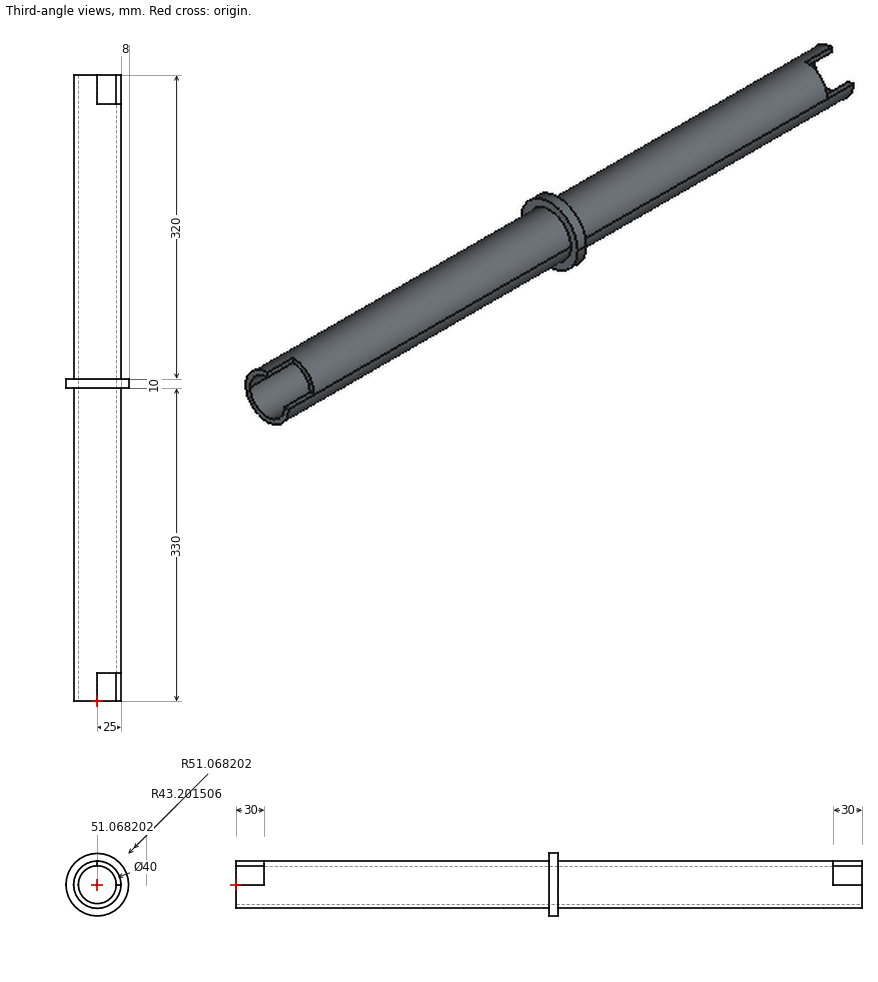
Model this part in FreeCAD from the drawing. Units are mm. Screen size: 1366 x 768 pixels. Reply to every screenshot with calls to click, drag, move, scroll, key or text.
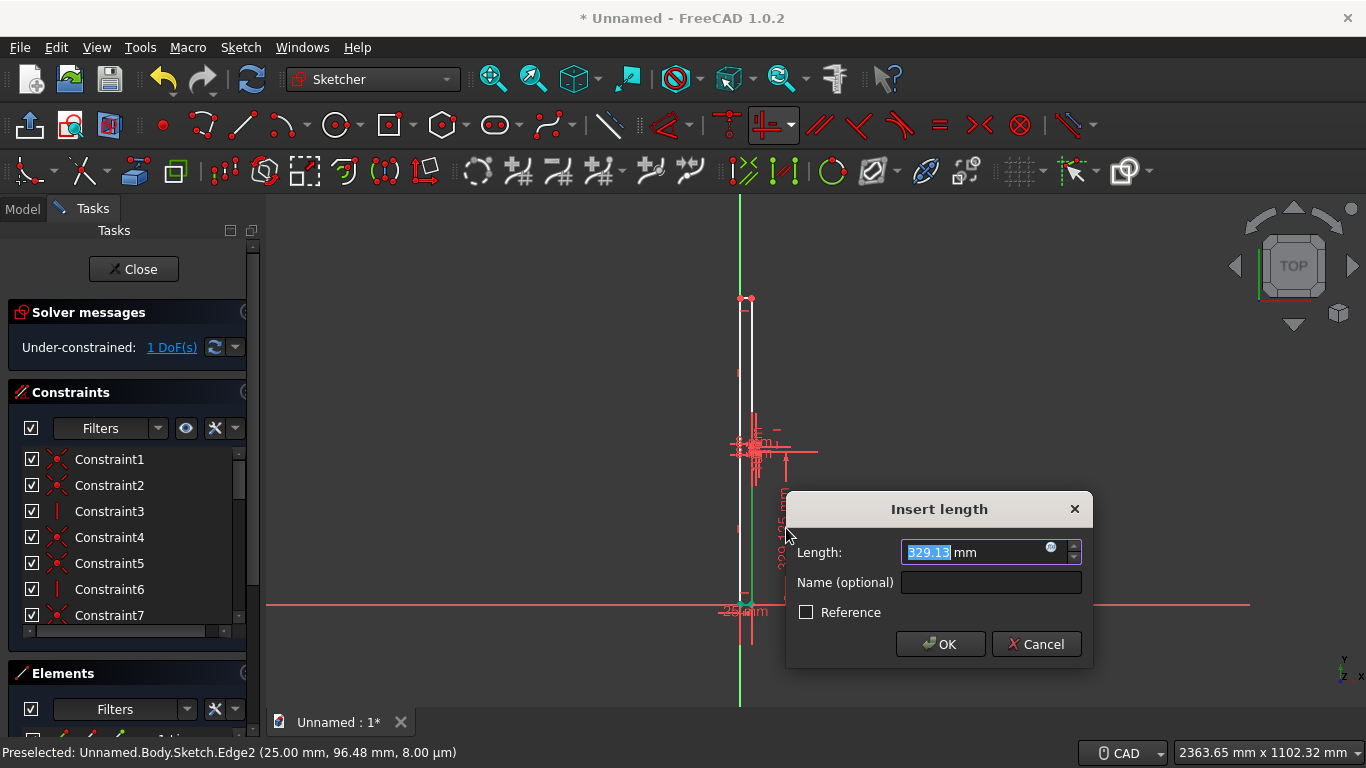
text(330)
key(Return)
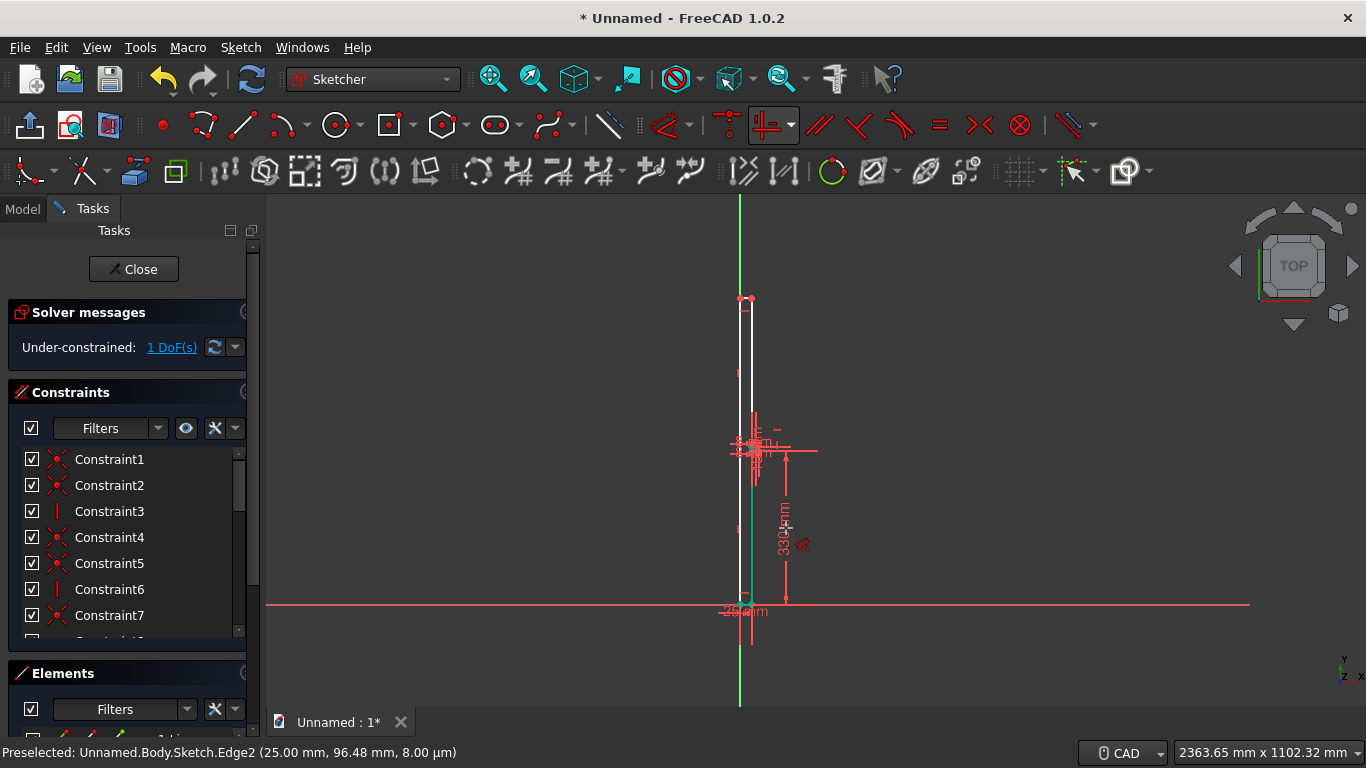
click(752, 402)
click(786, 372)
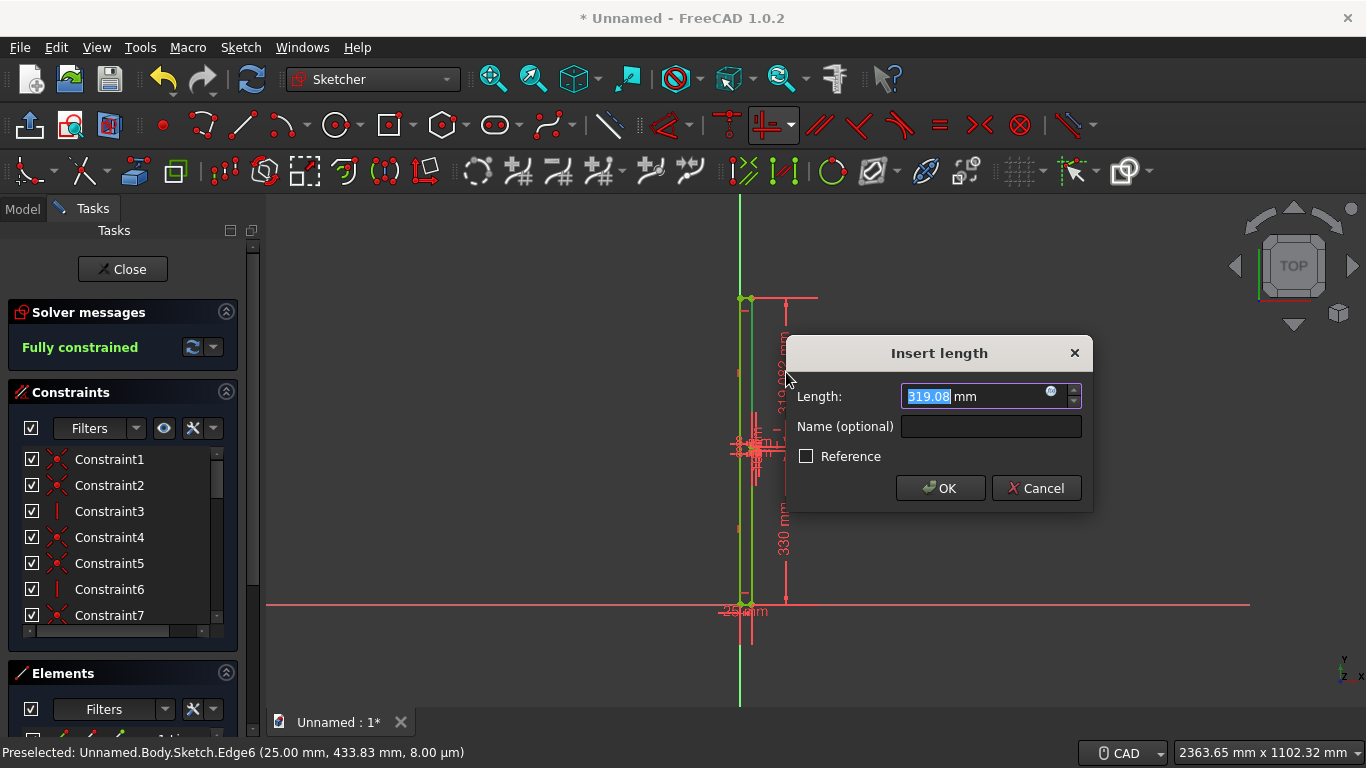
text(320)
key(Return)
key(Escape)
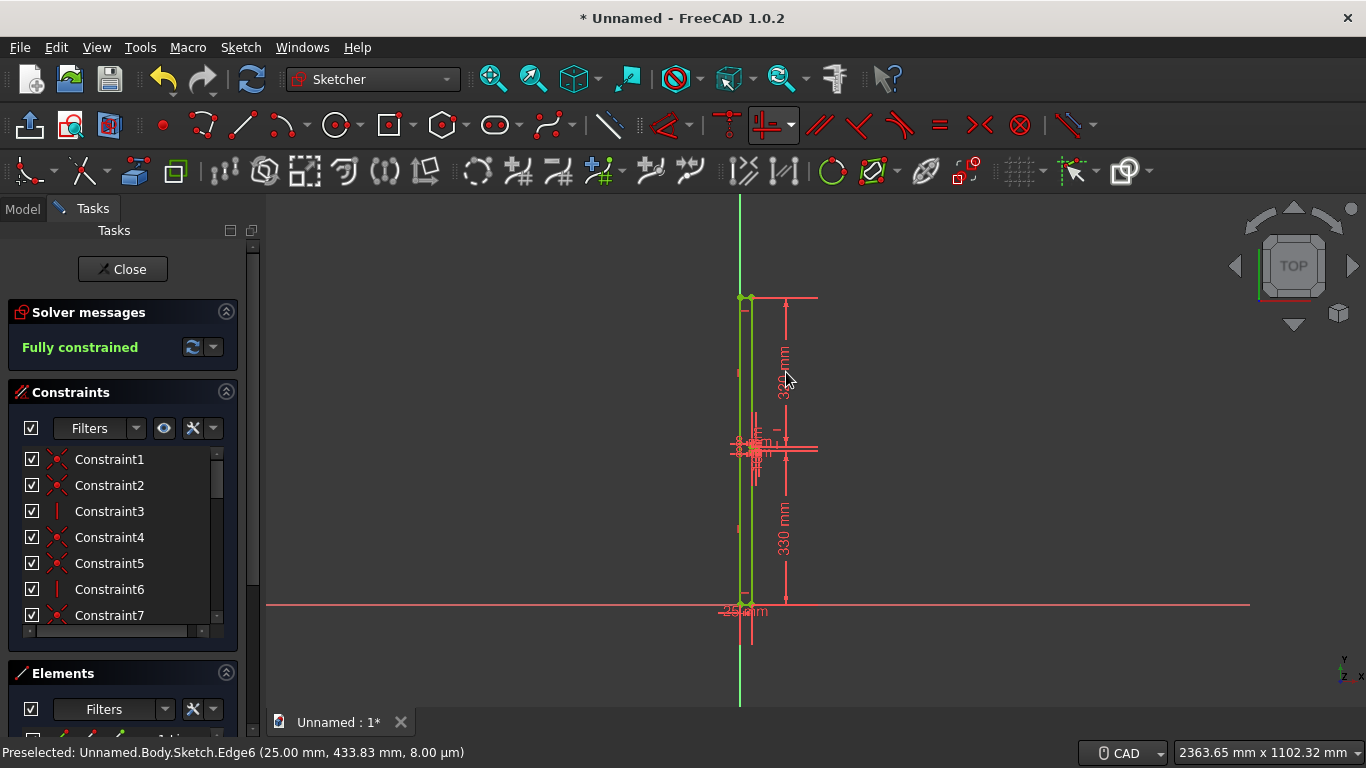
click(123, 269)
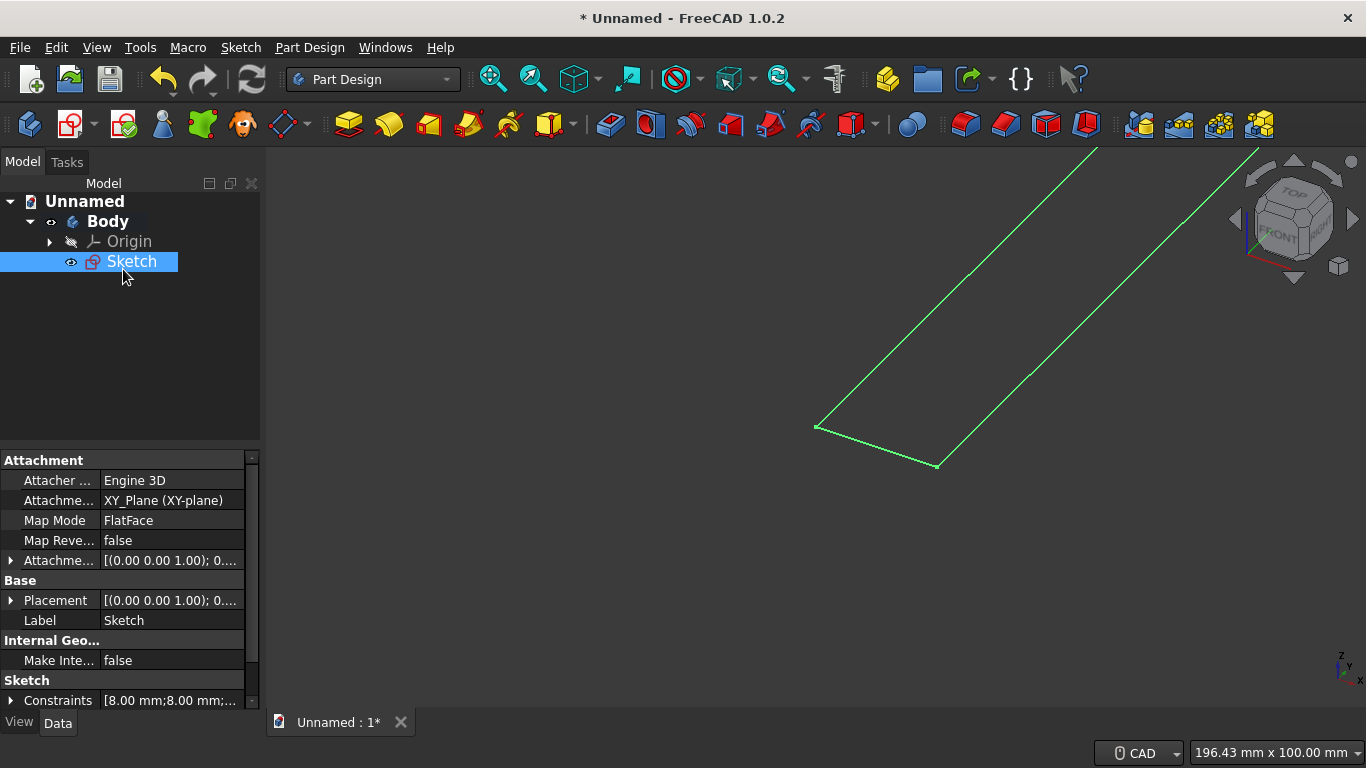
click(390, 124)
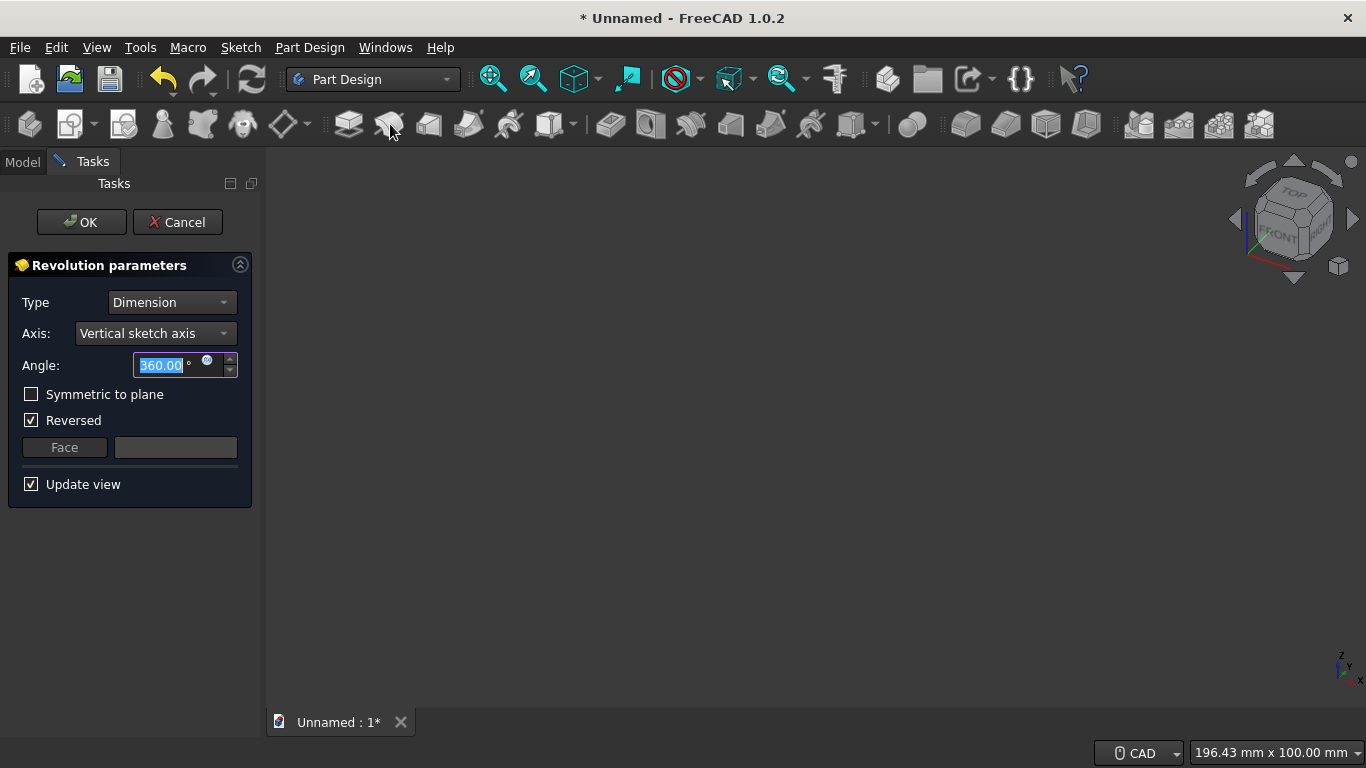
click(82, 222)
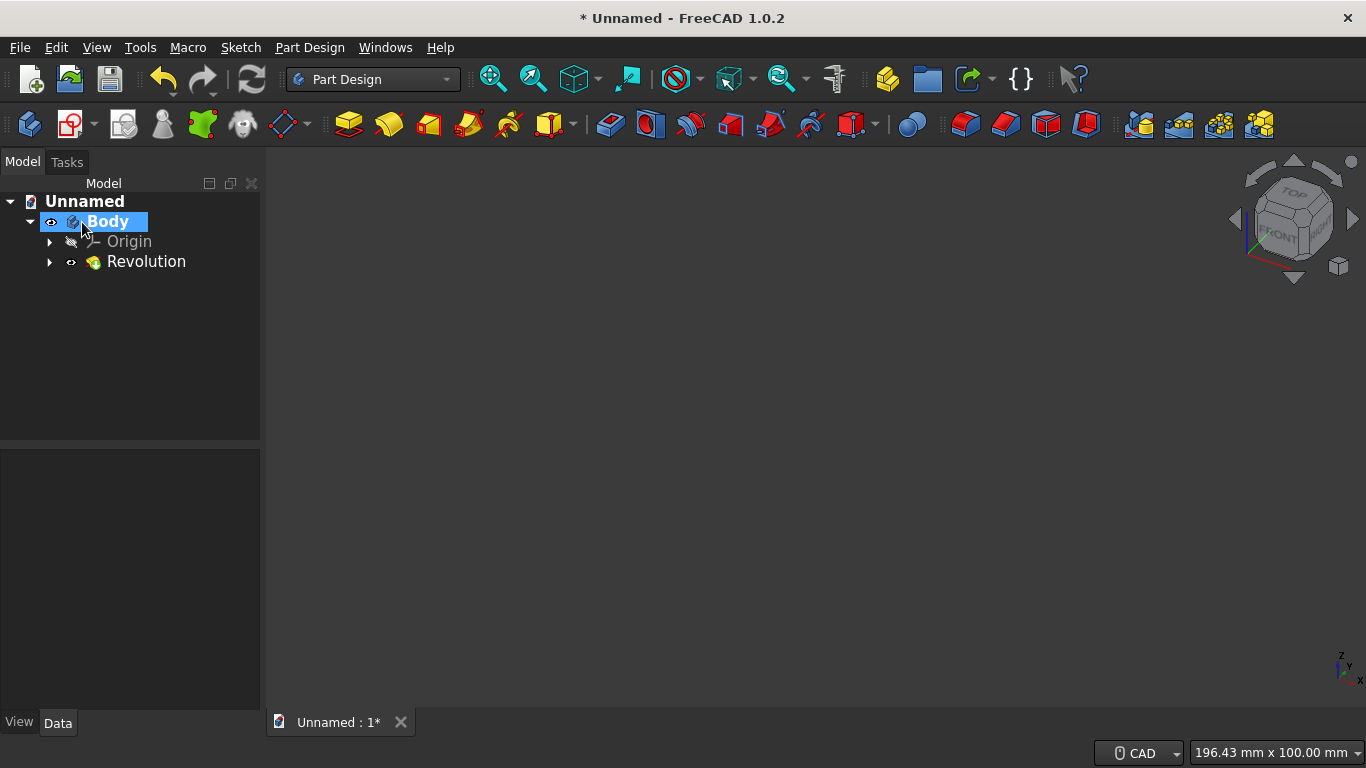
click(494, 80)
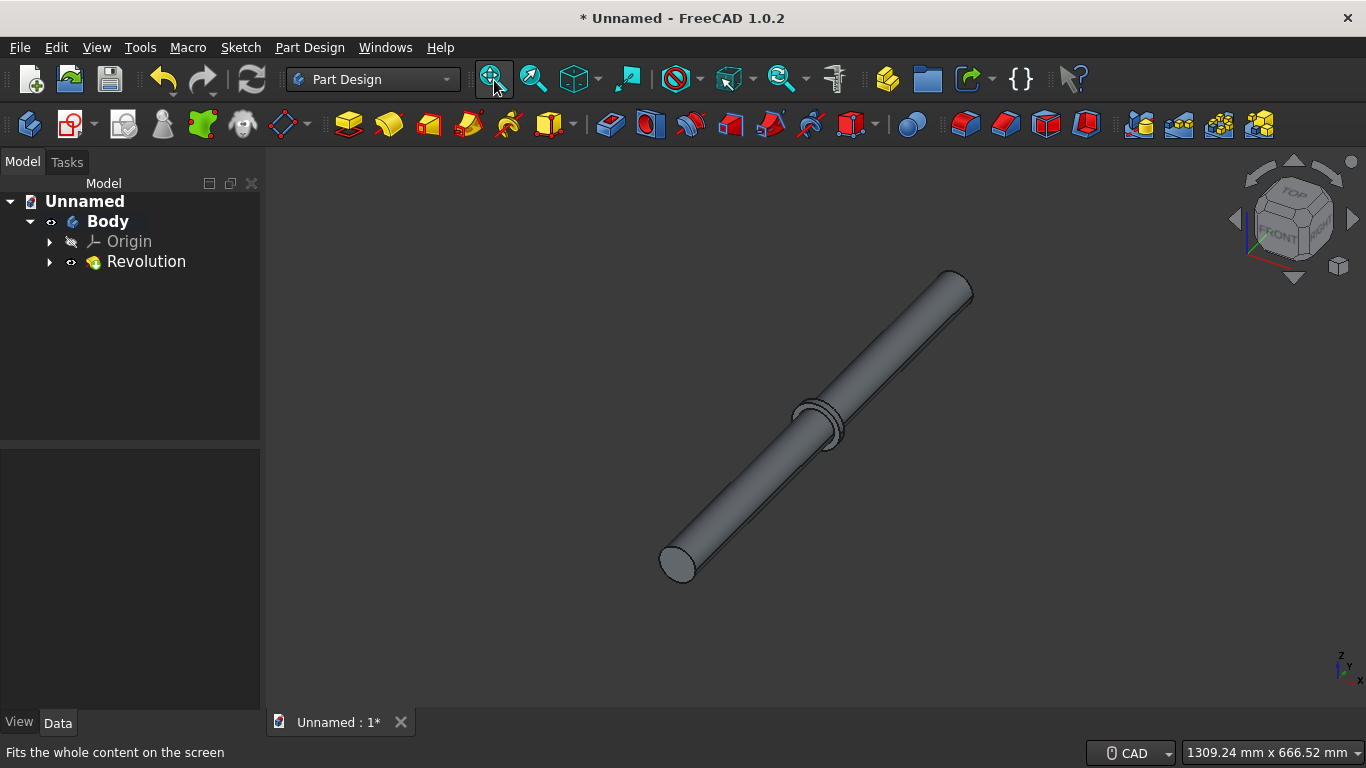
key(4)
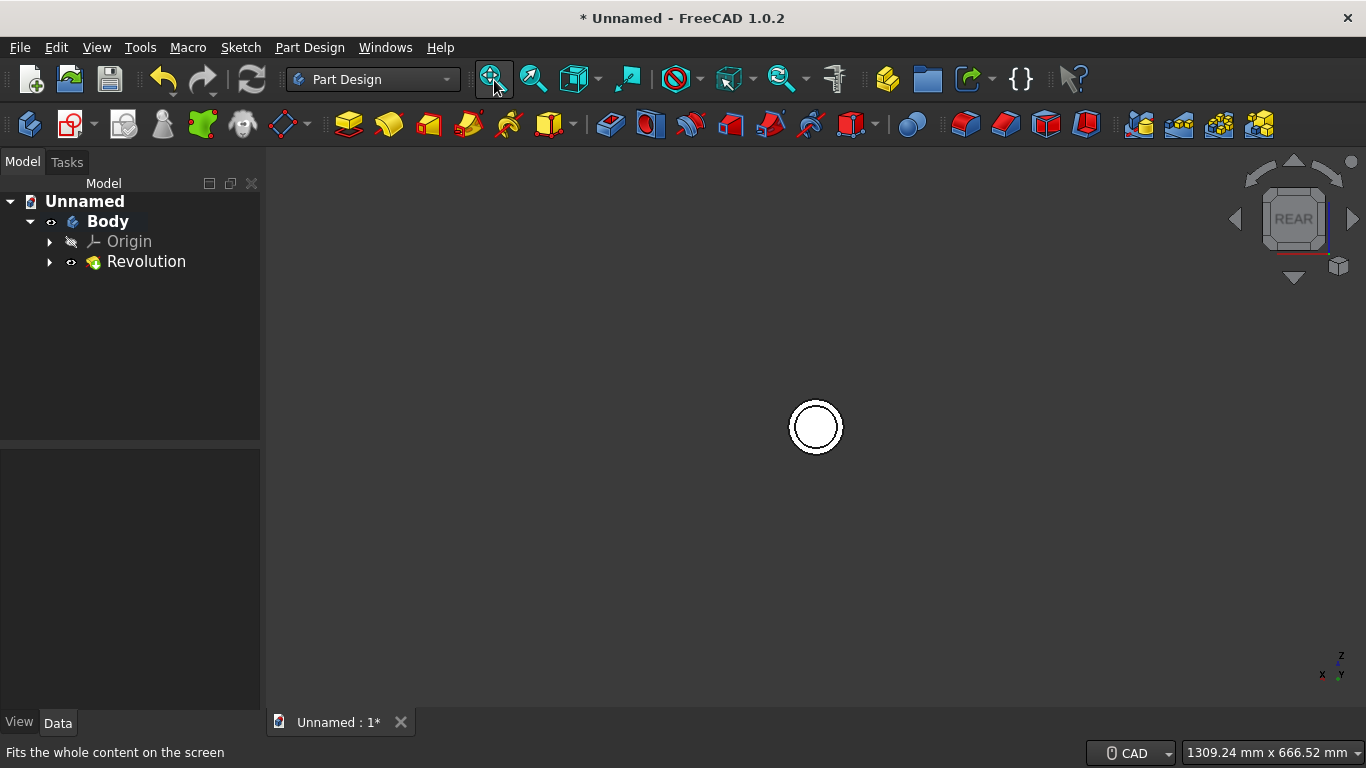
click(494, 80)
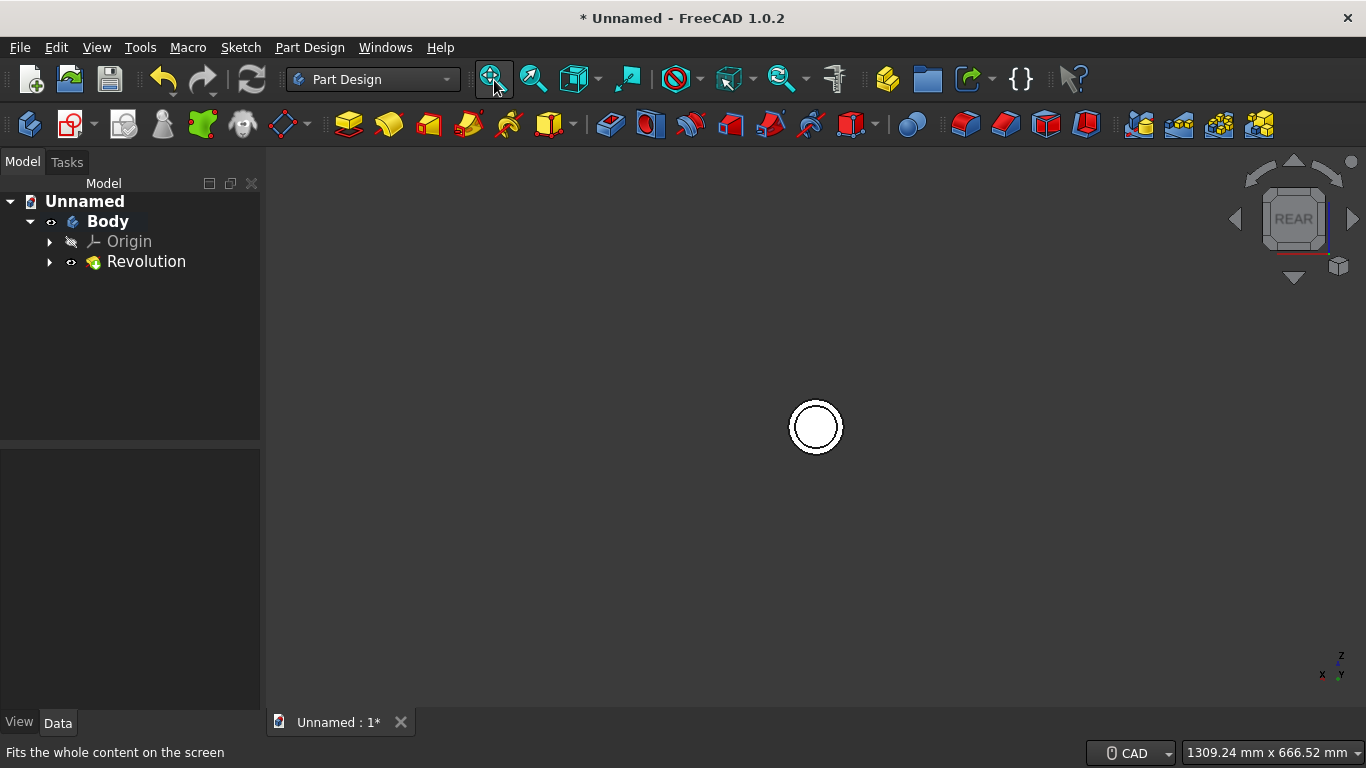
click(816, 426)